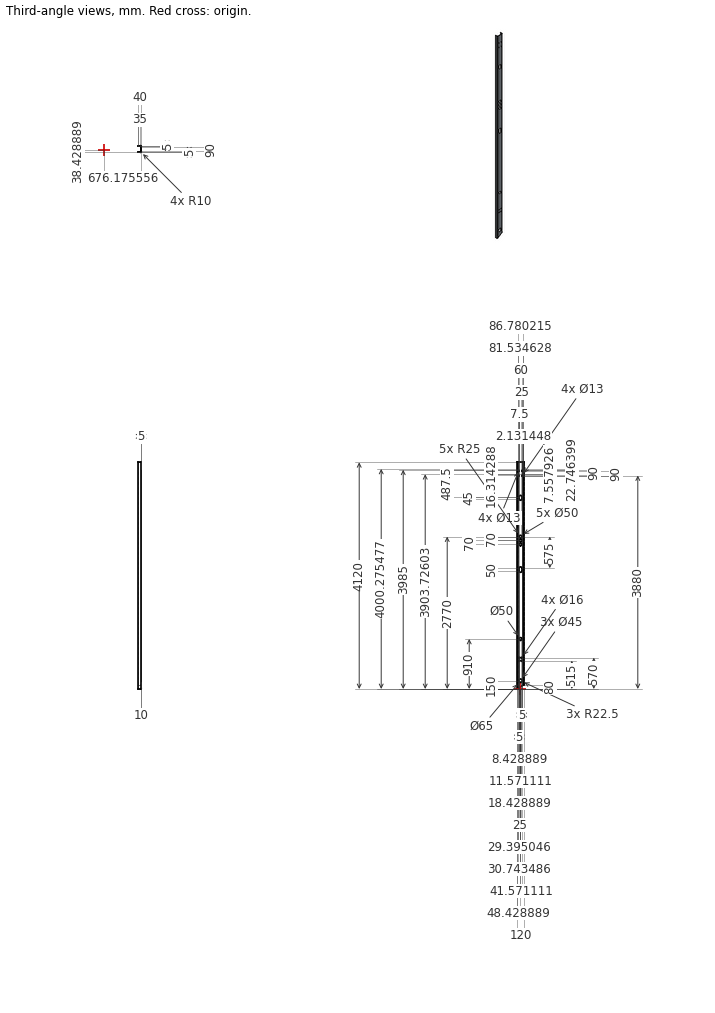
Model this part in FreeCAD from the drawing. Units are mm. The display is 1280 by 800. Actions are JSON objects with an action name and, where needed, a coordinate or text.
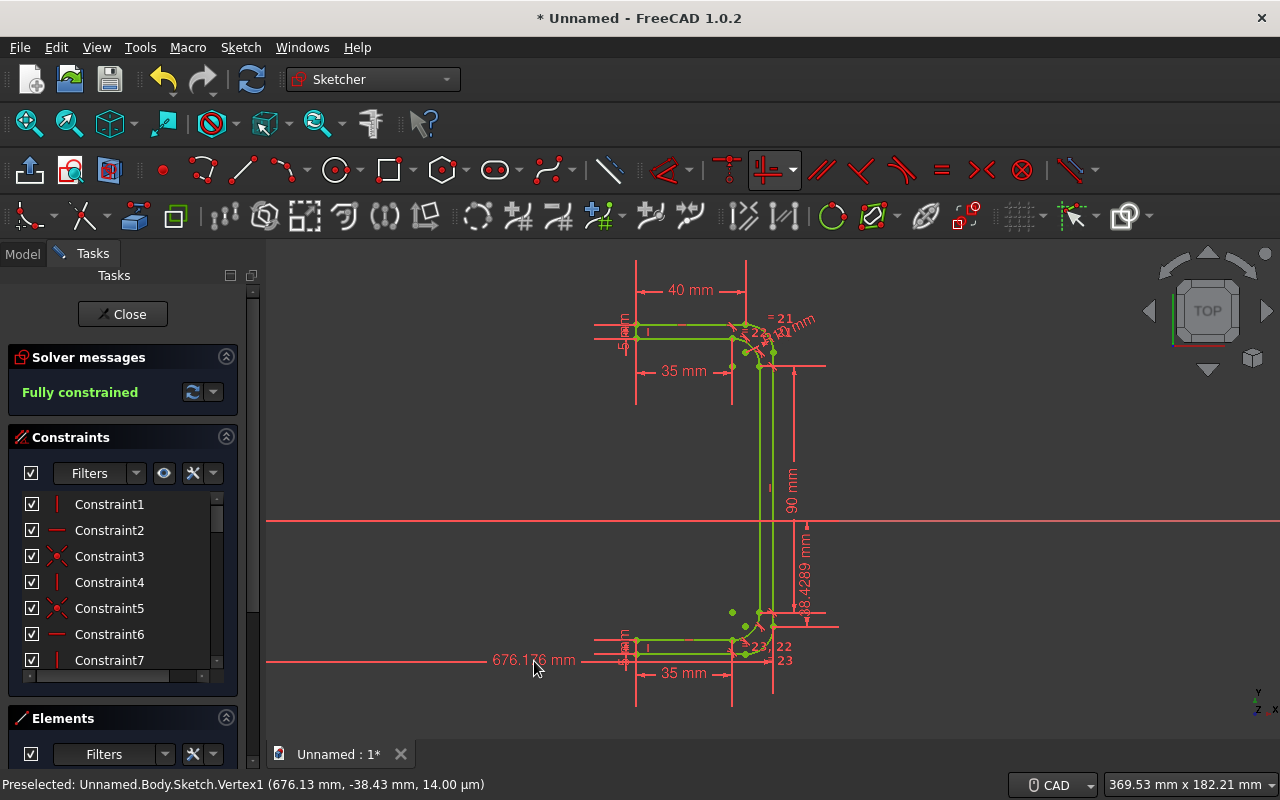
{"action": "left_click", "coordinate": [123, 314]}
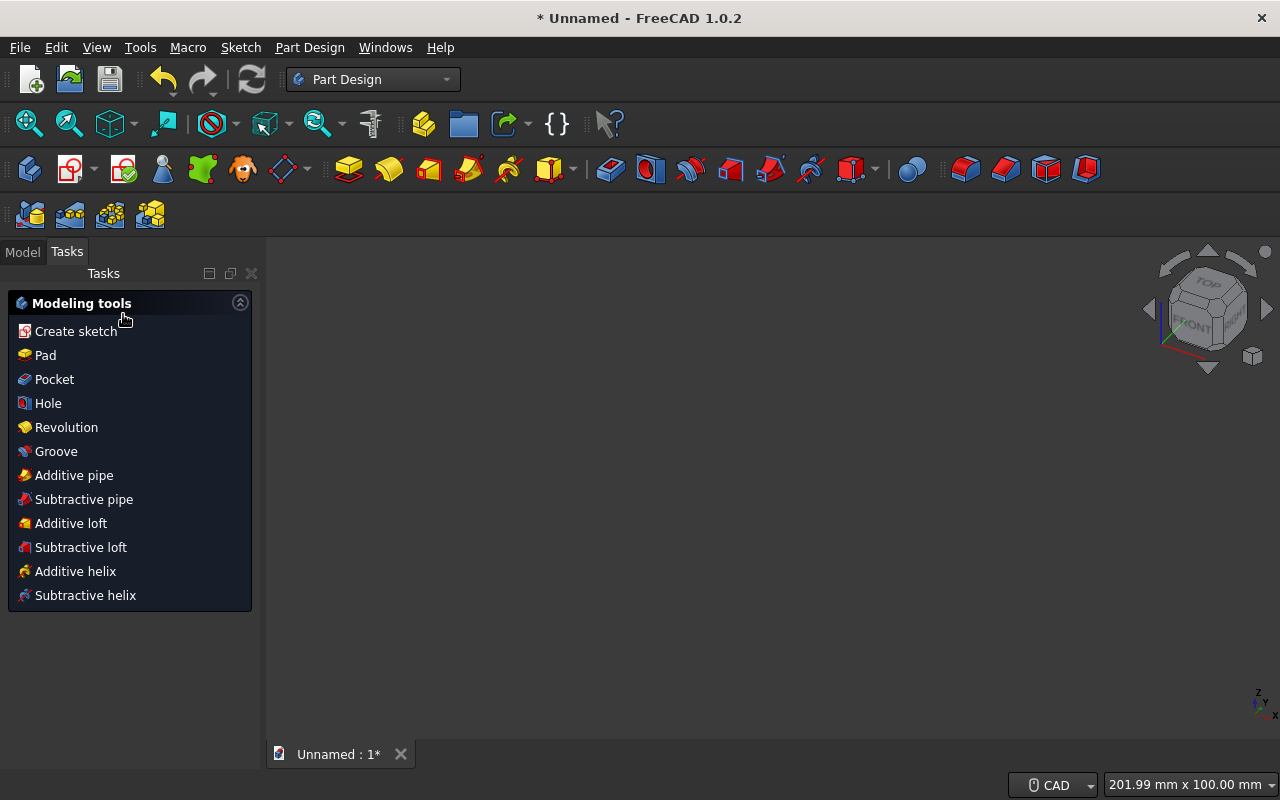
{"action": "left_click", "coordinate": [350, 170]}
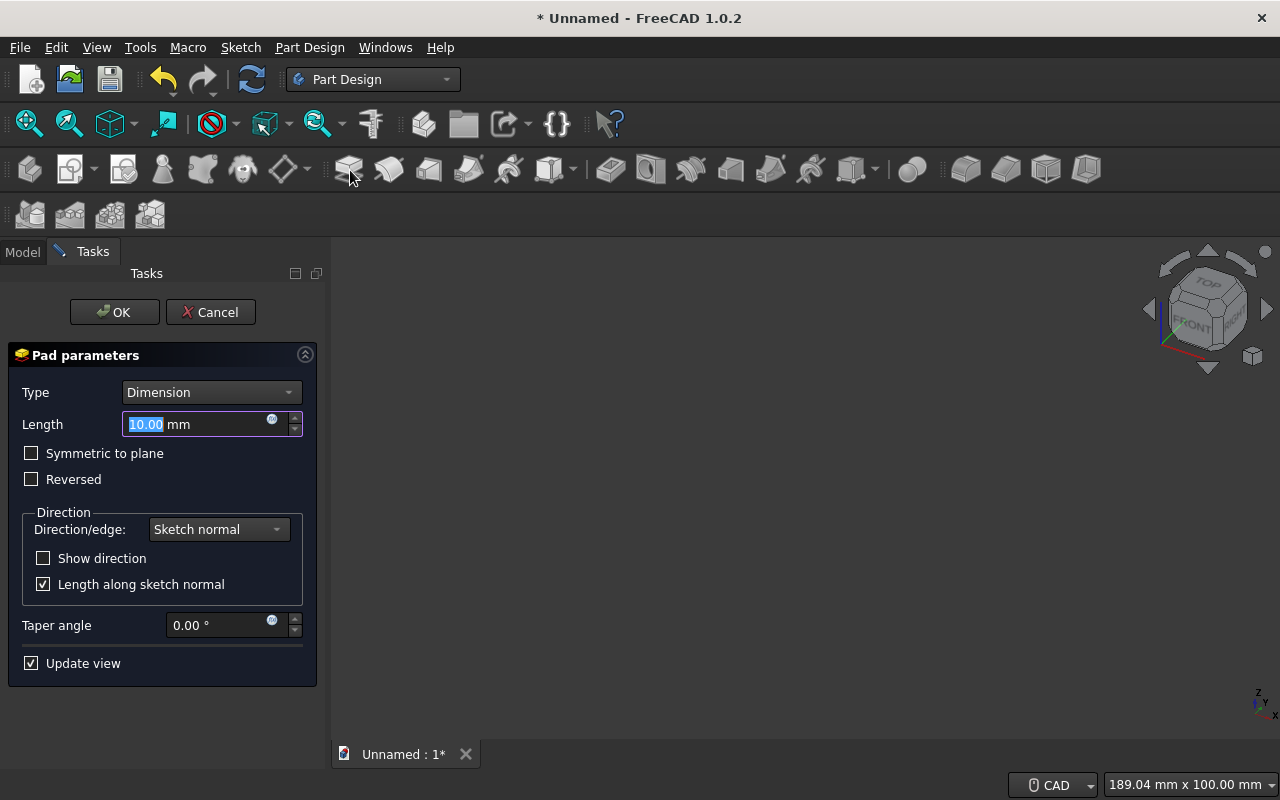
{"action": "type", "text": "4120"}
{"action": "key", "text": "Tab"}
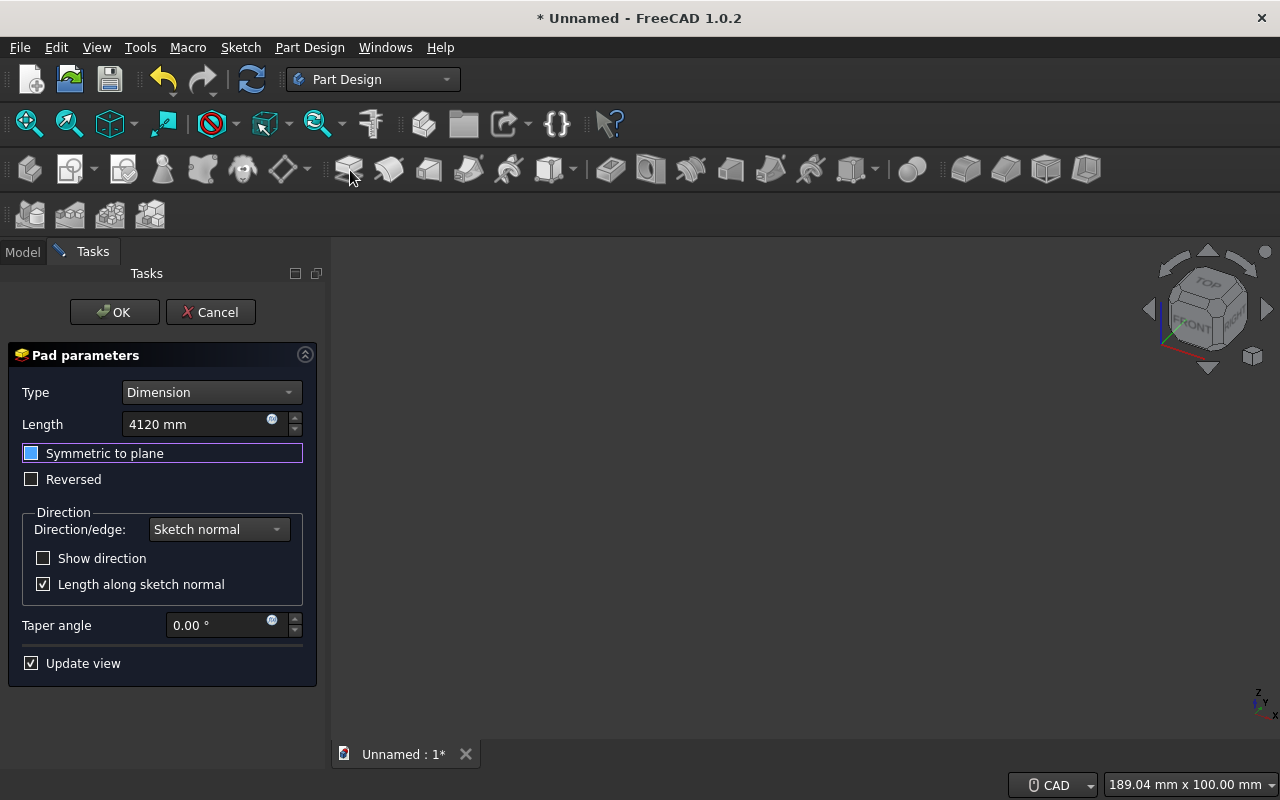
{"action": "left_click", "coordinate": [115, 312]}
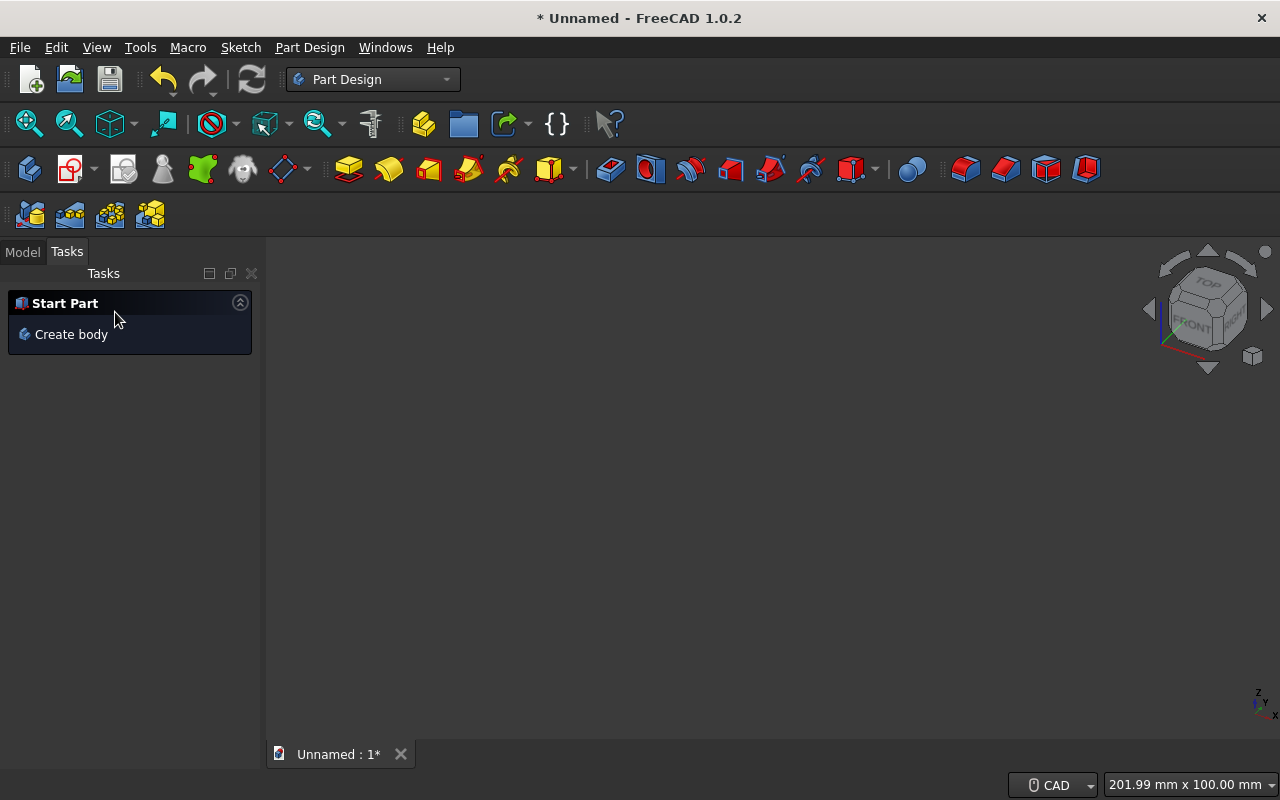
{"action": "key", "text": "v f"}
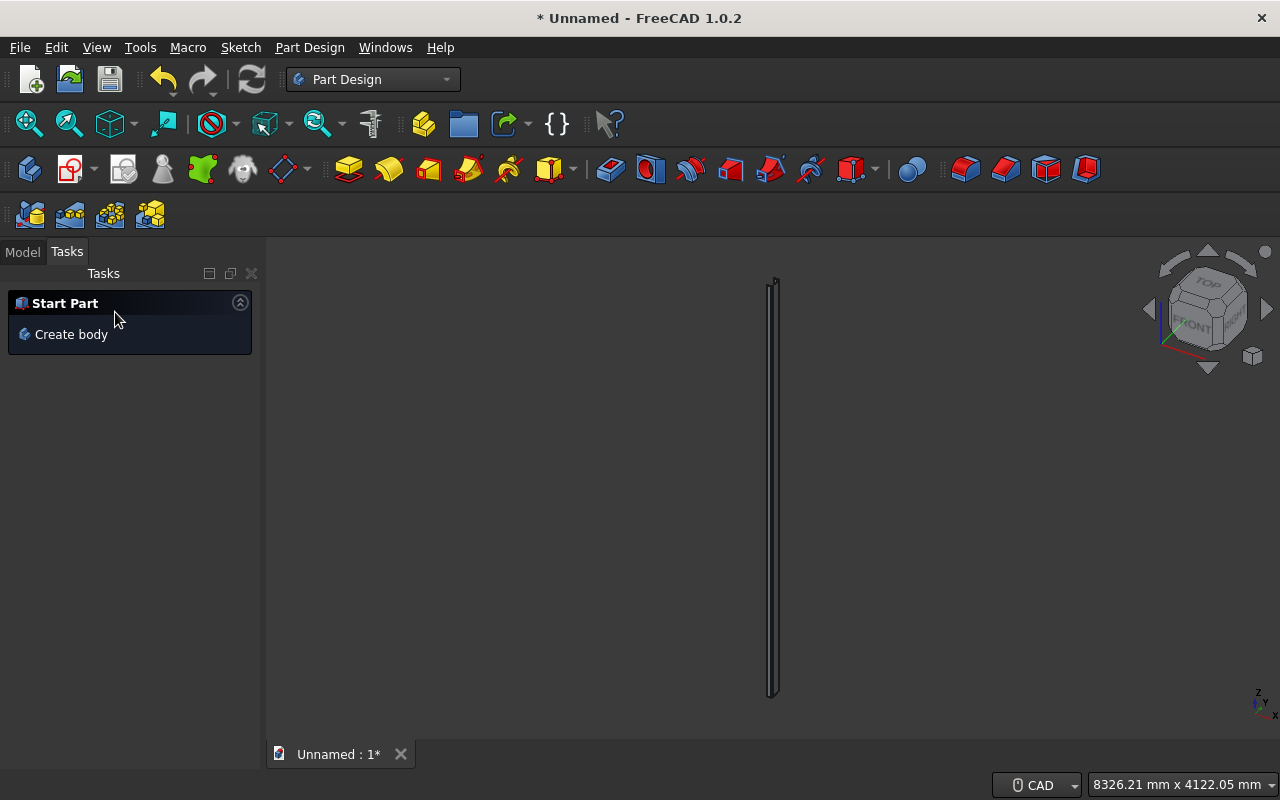
{"action": "scroll", "coordinate": [776, 312], "scroll_direction": "up", "scroll_amount": 4}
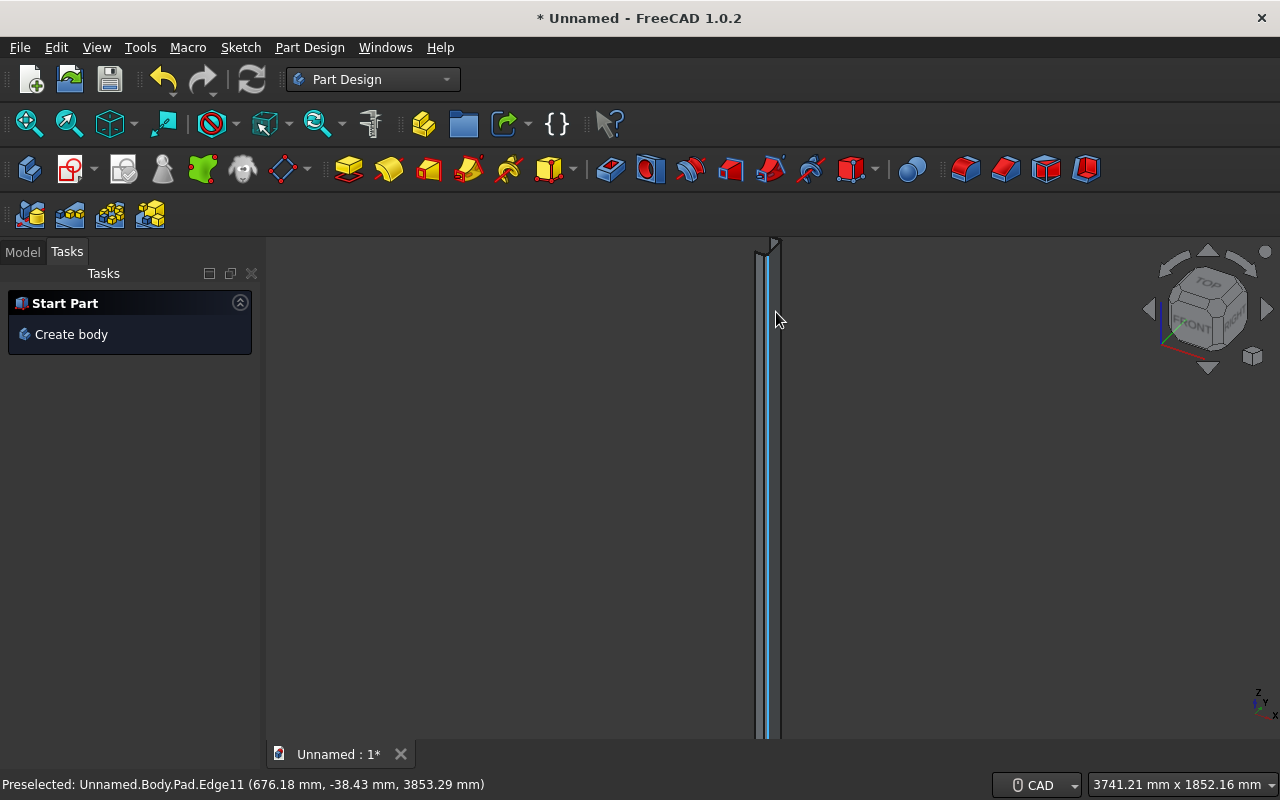
{"action": "key", "text": "v f"}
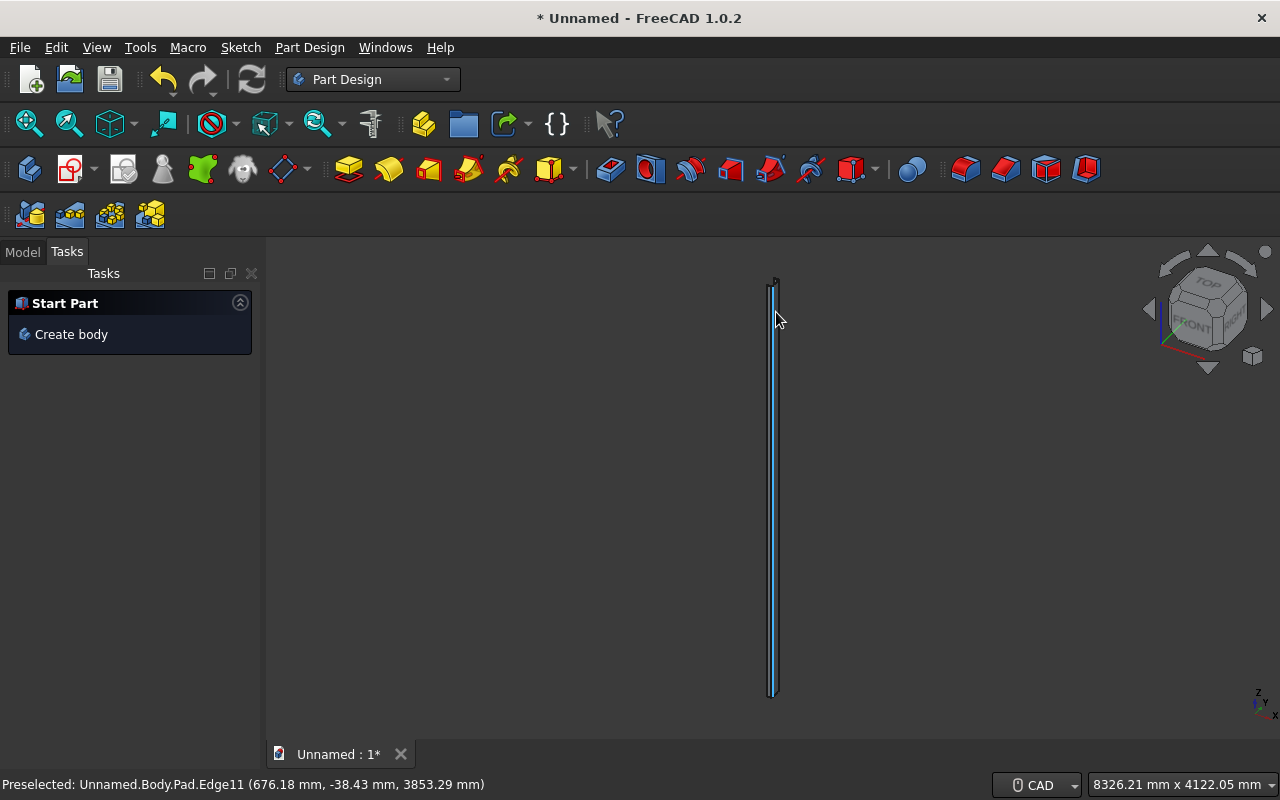
{"action": "key", "text": "0"}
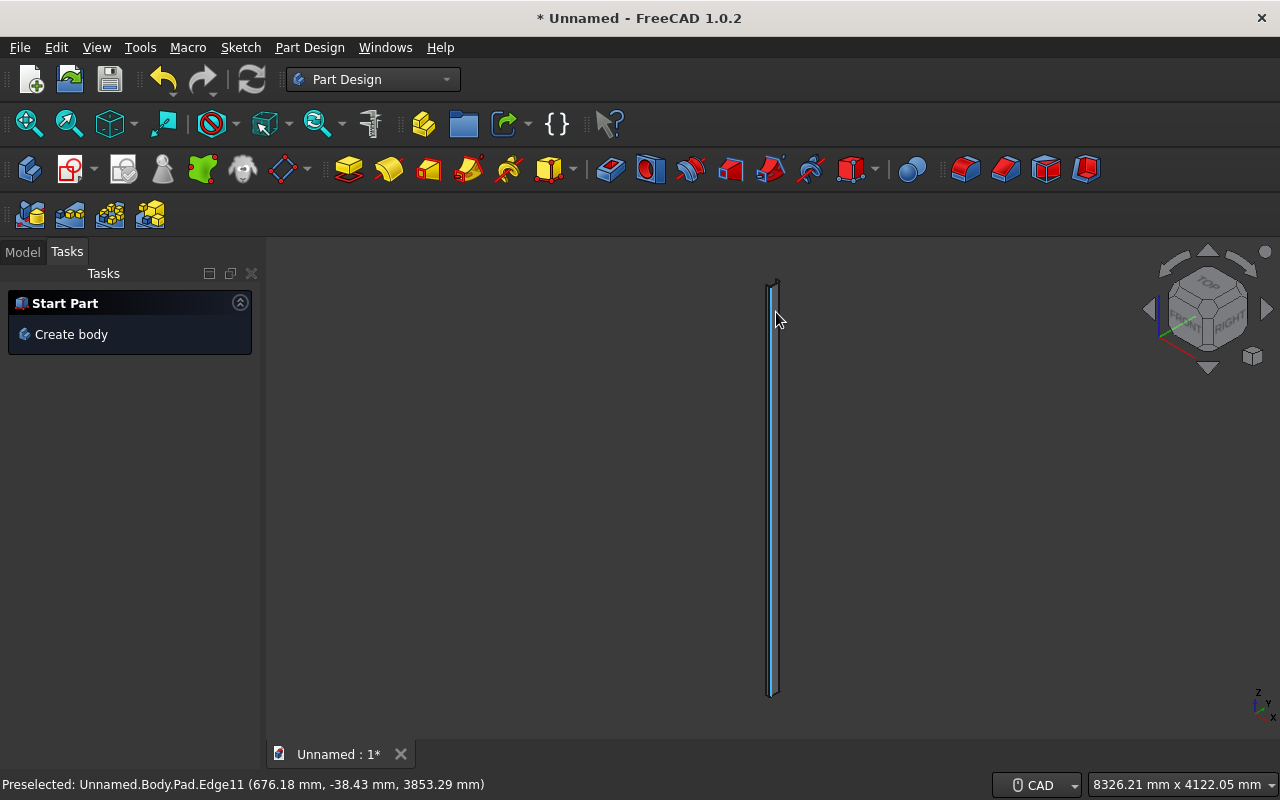
{"action": "scroll", "coordinate": [775, 313], "scroll_direction": "up", "scroll_amount": 4}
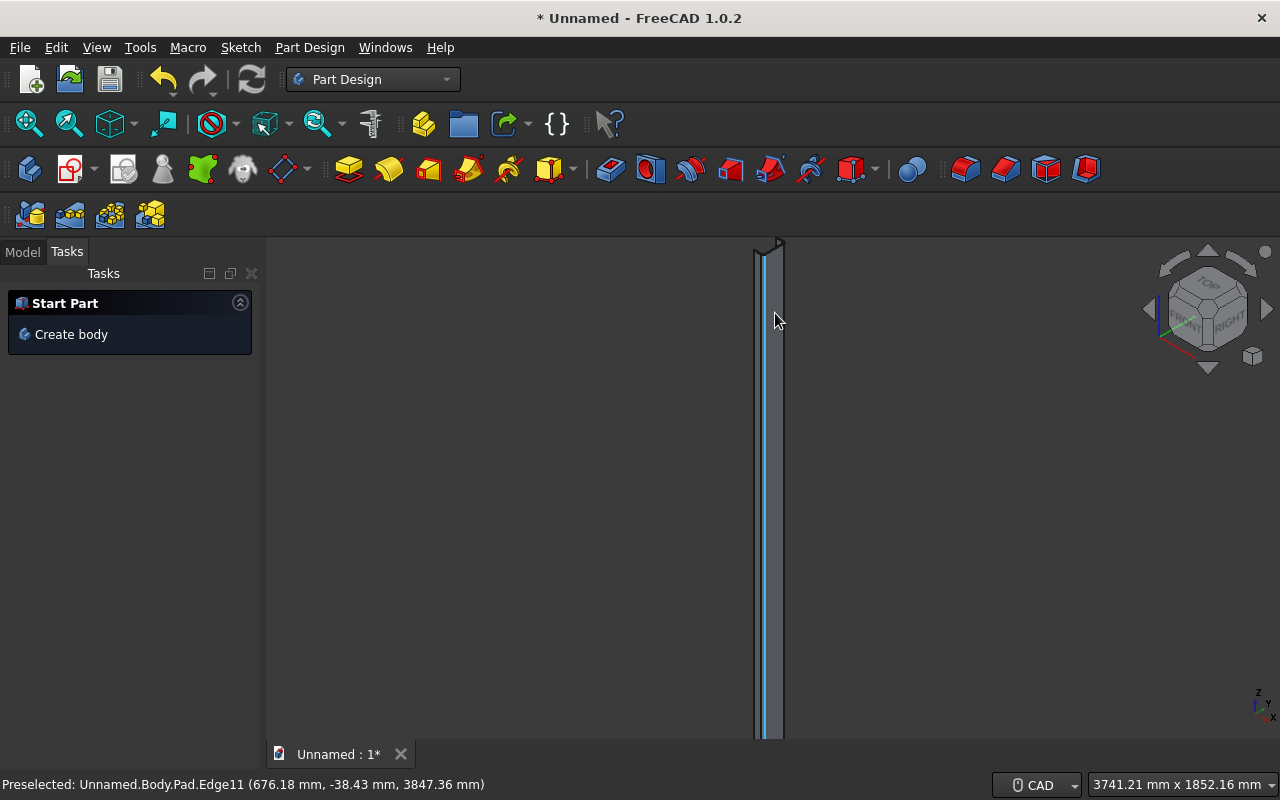
{"action": "left_click", "coordinate": [775, 313]}